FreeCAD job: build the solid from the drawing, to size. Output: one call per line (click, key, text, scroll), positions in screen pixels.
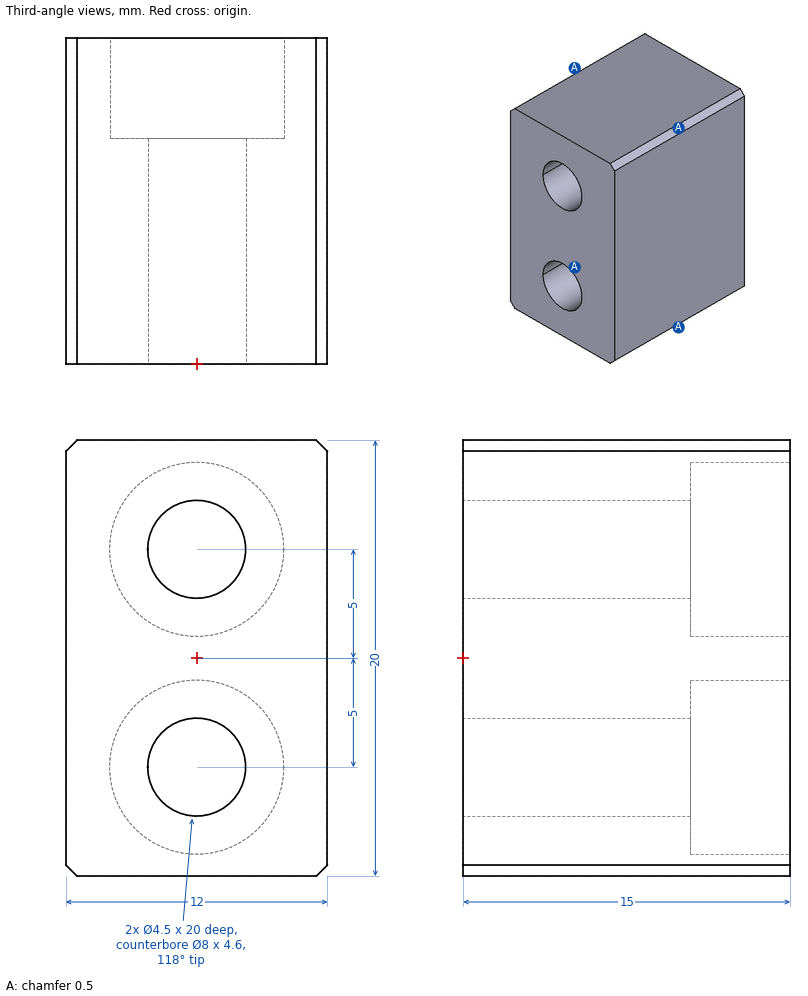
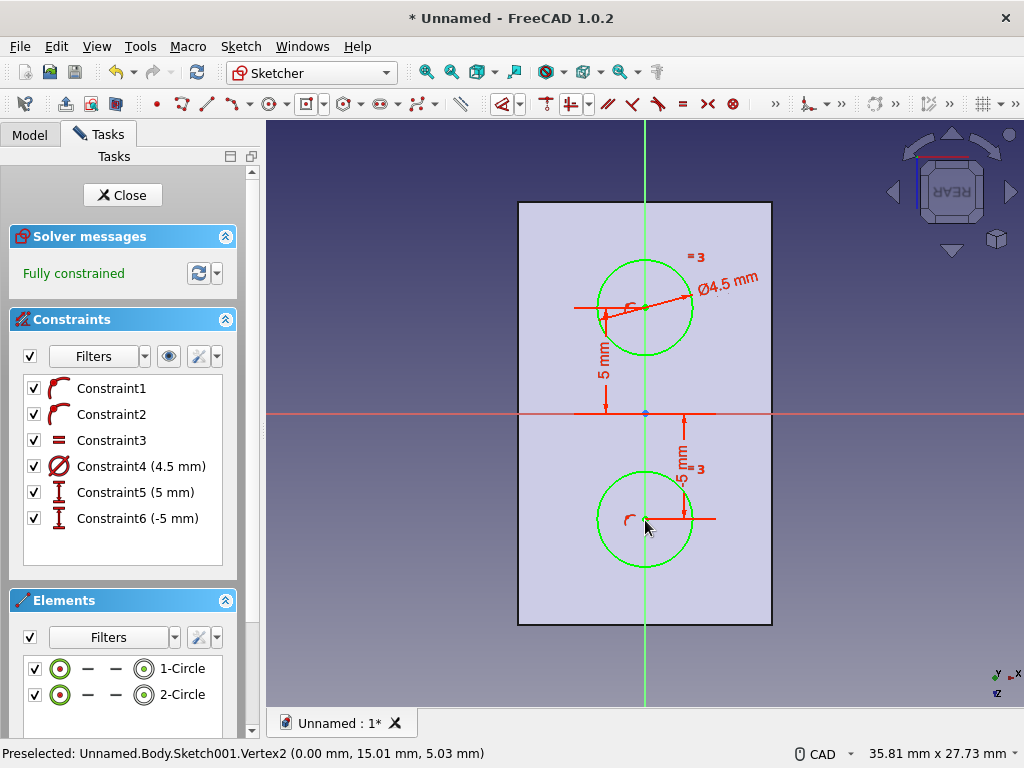
click(123, 195)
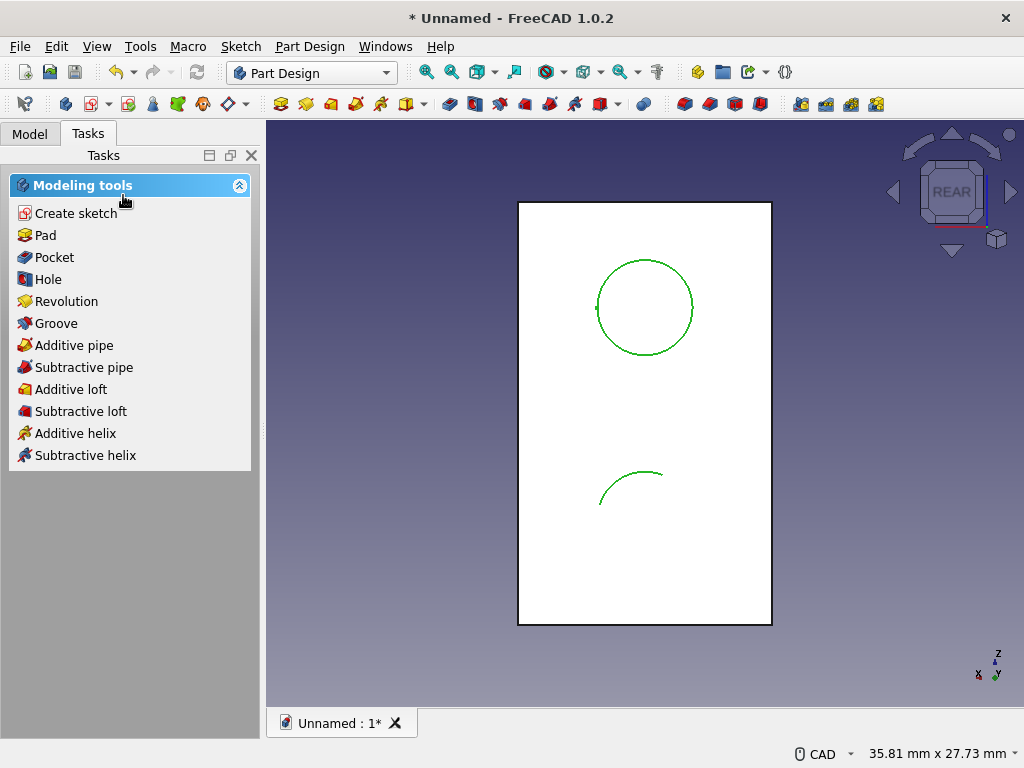
click(475, 104)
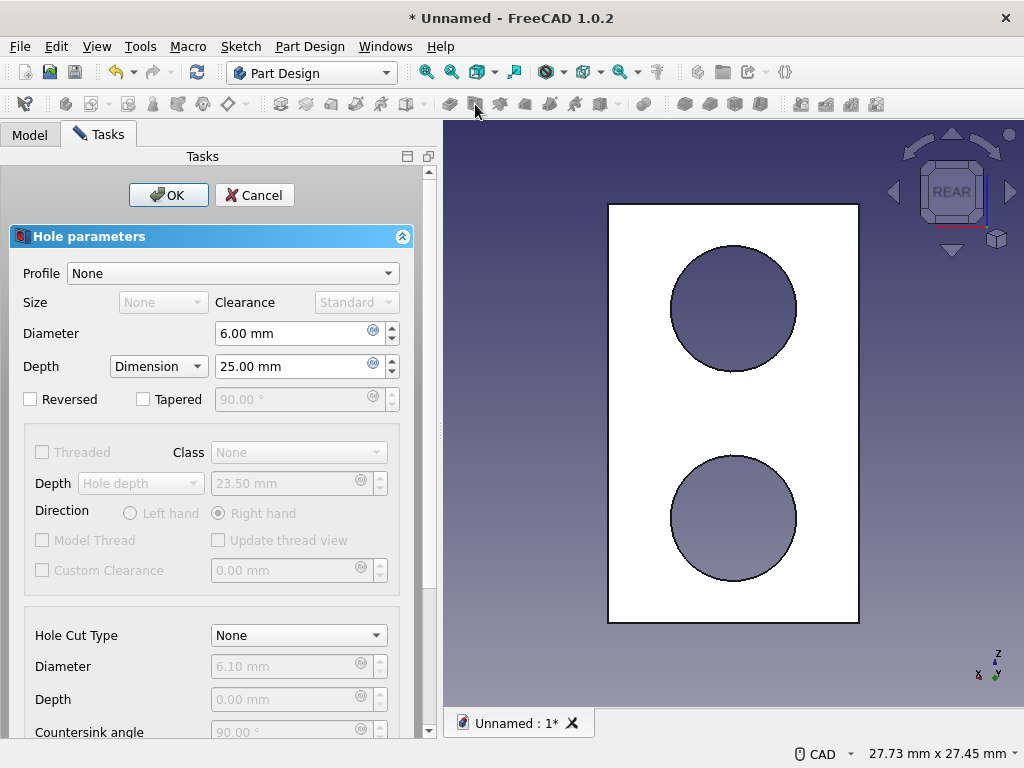
triple_click(300, 334)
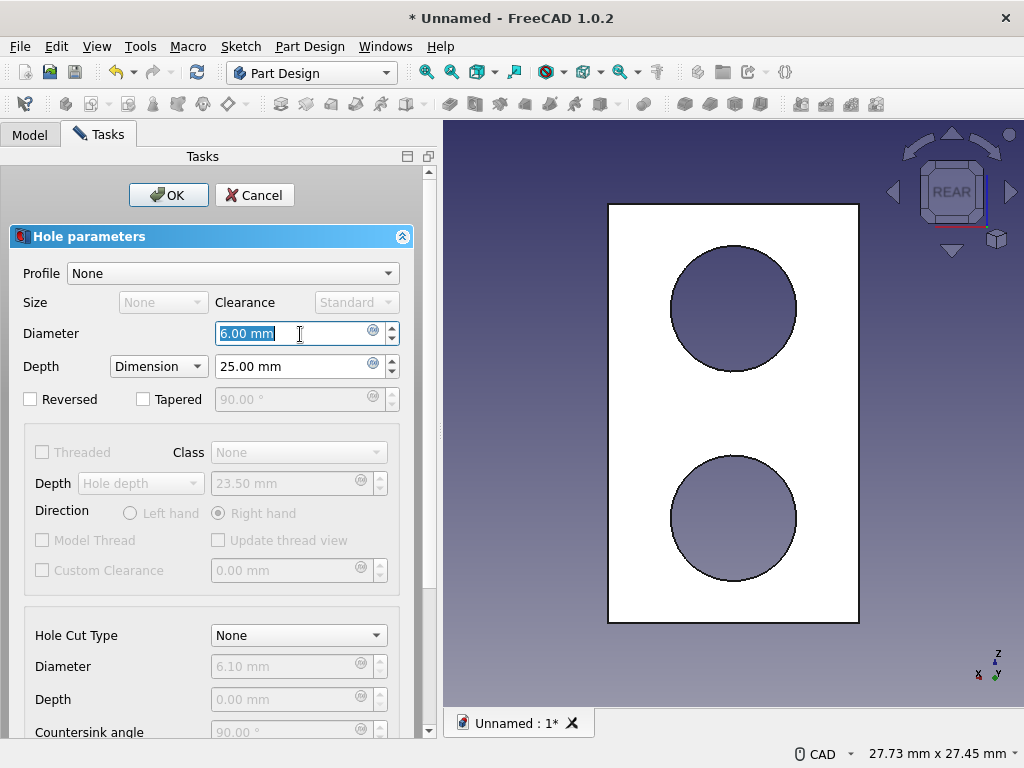
text(4.5)
key(Tab)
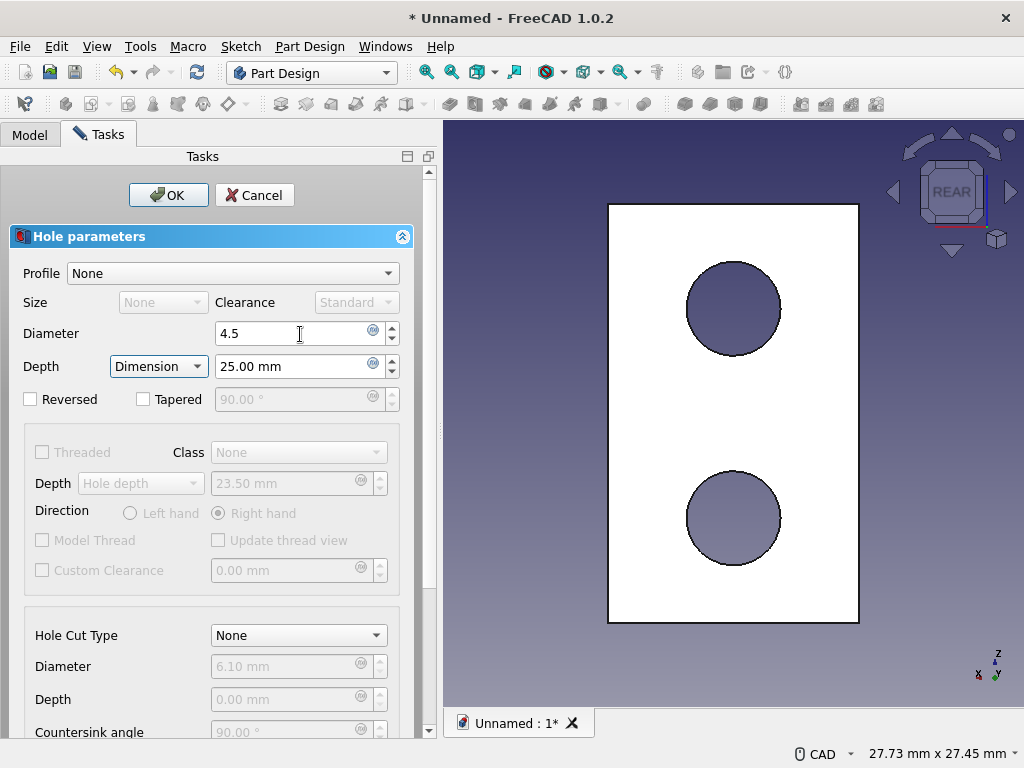
triple_click(300, 366)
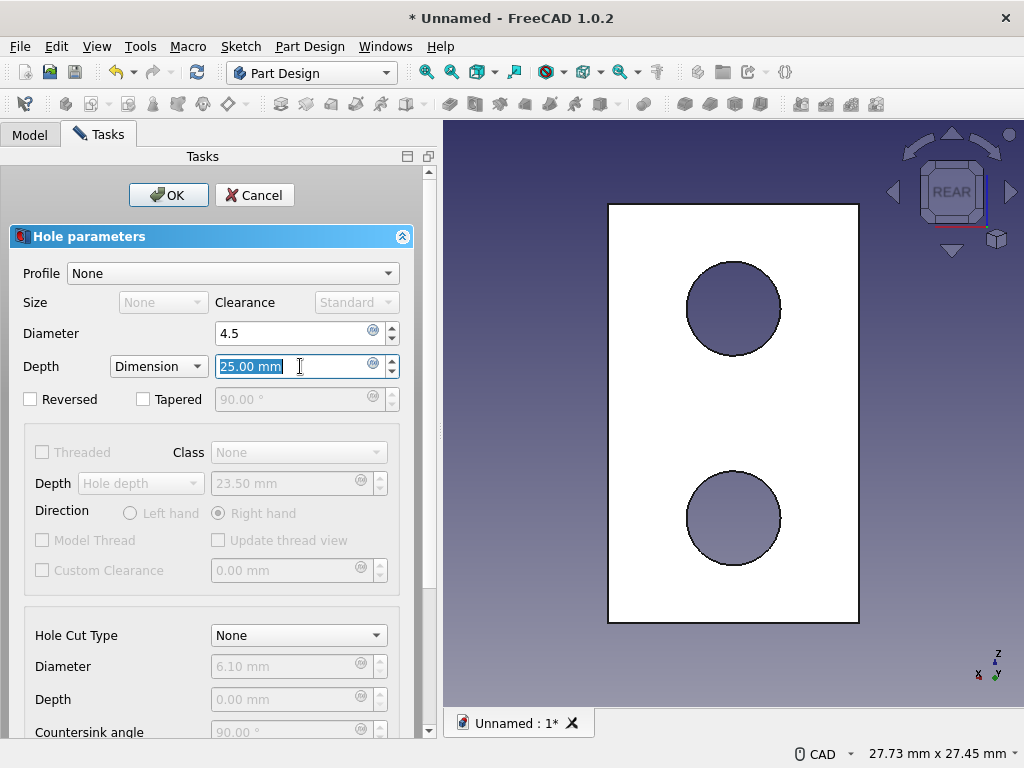
text(20)
key(Tab)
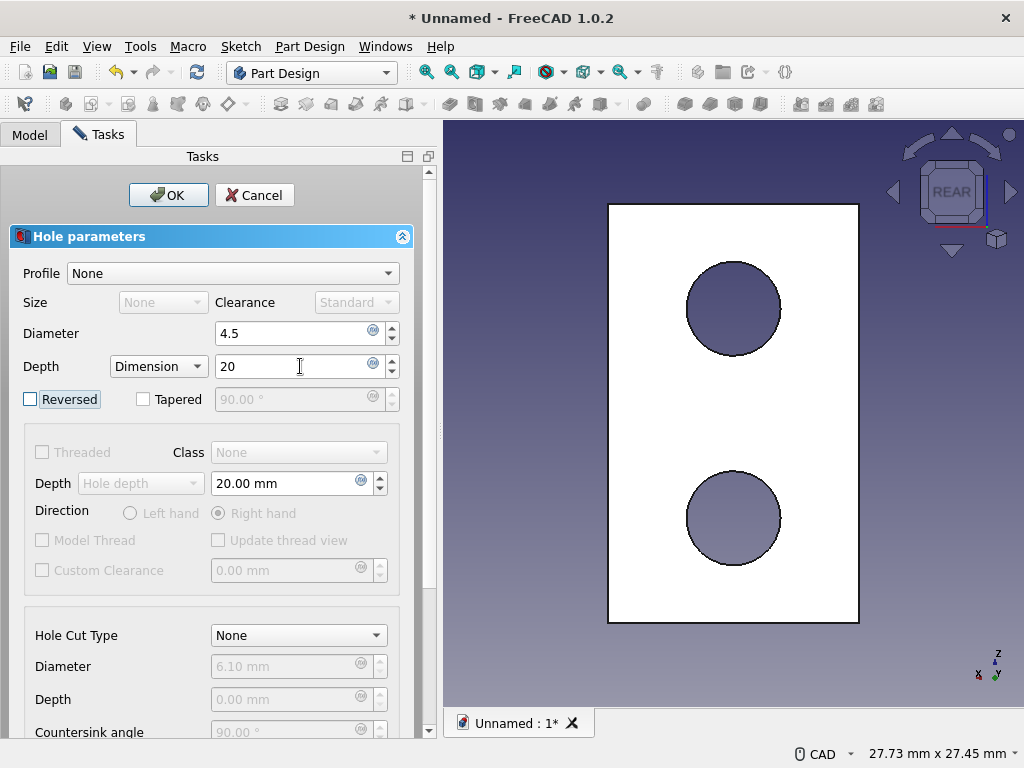
click(300, 636)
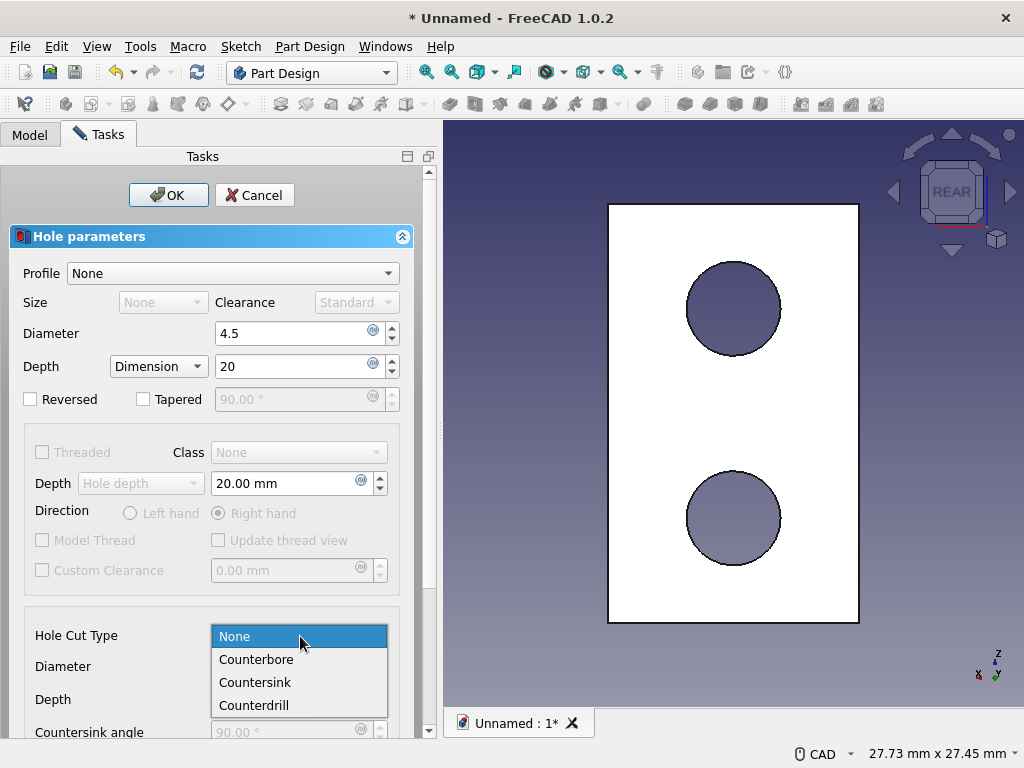
click(298, 660)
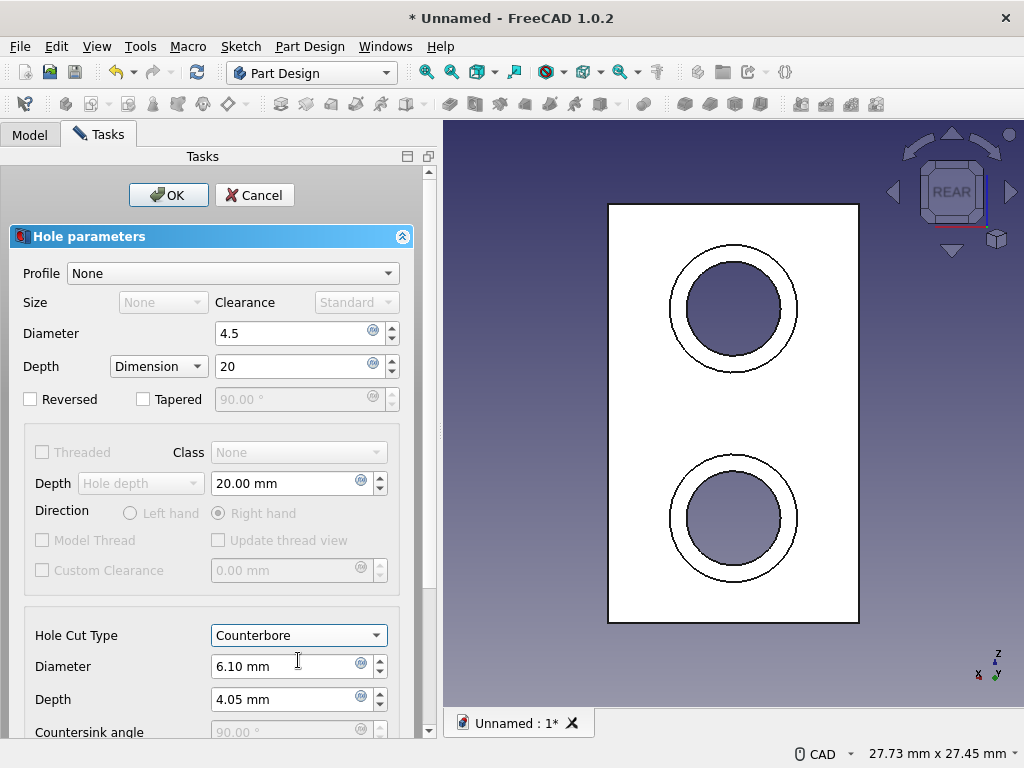
triple_click(292, 666)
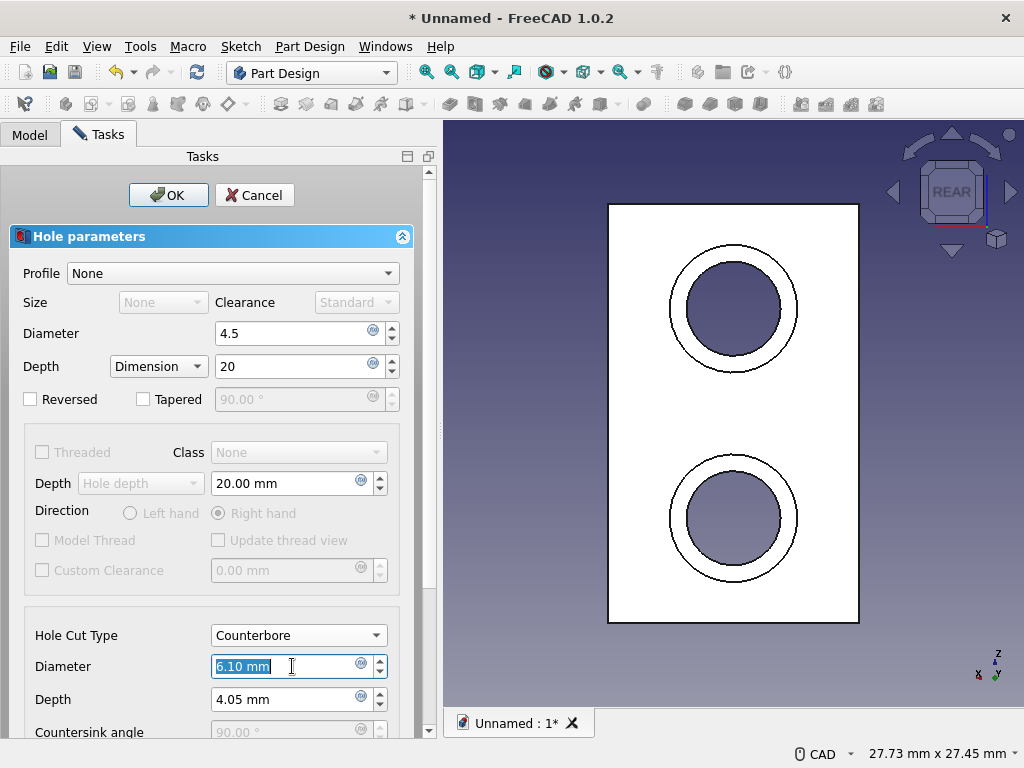
text(8)
key(Tab)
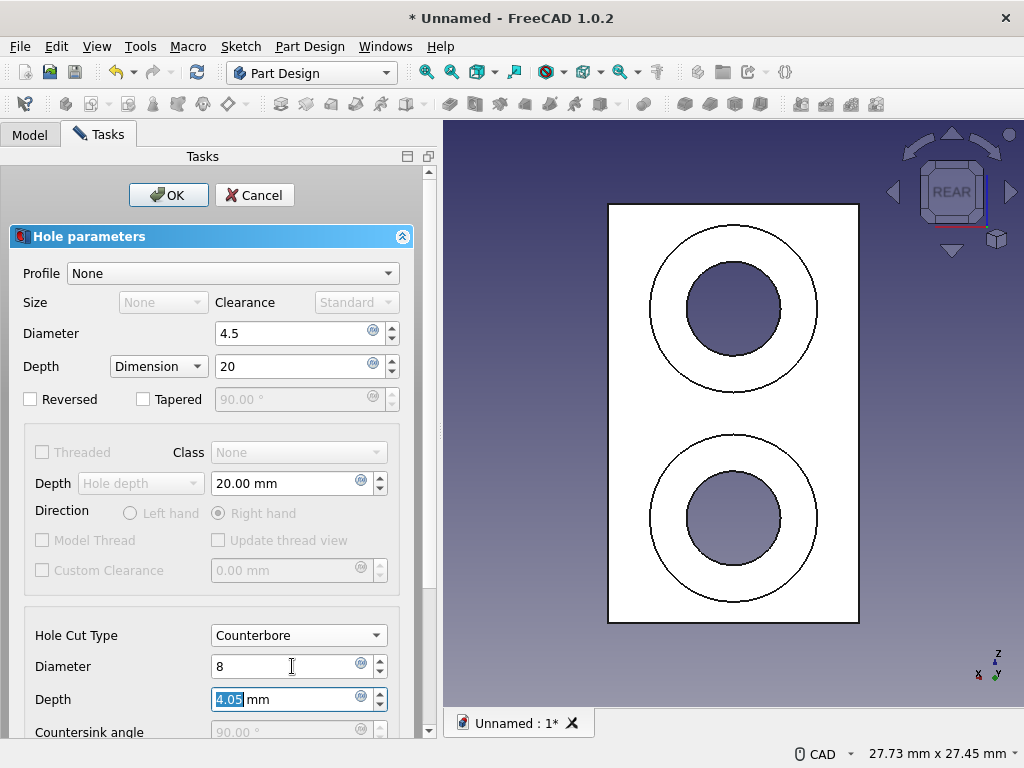
text(4.6)
key(Tab)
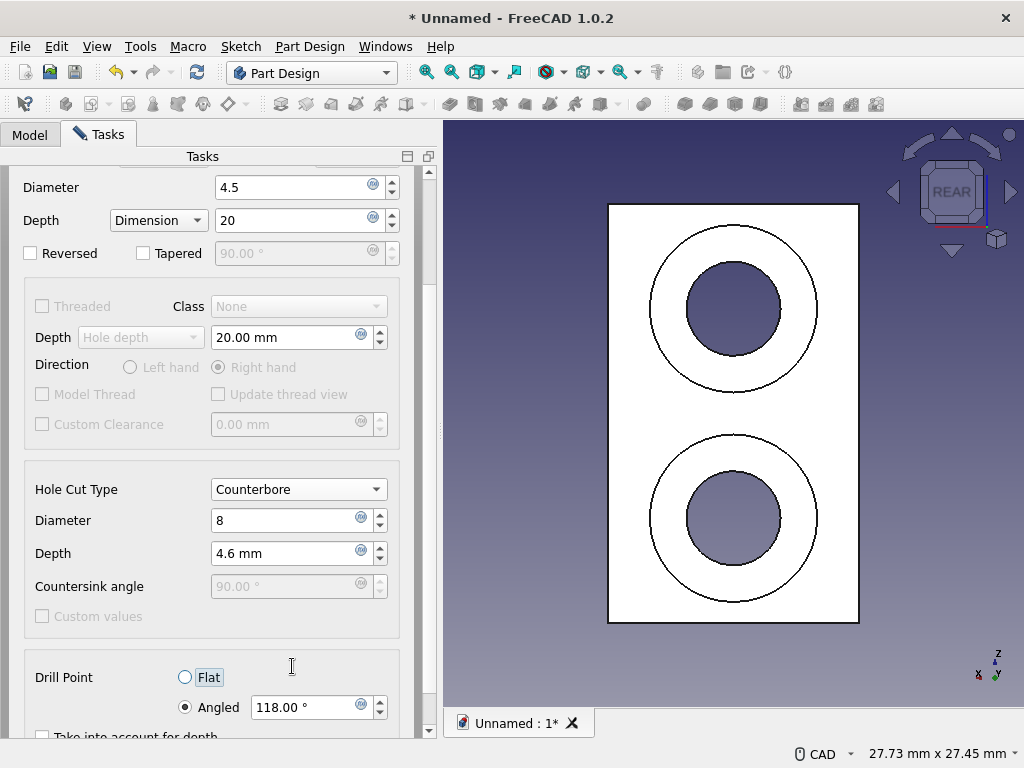
scroll(429, 452, up, 4)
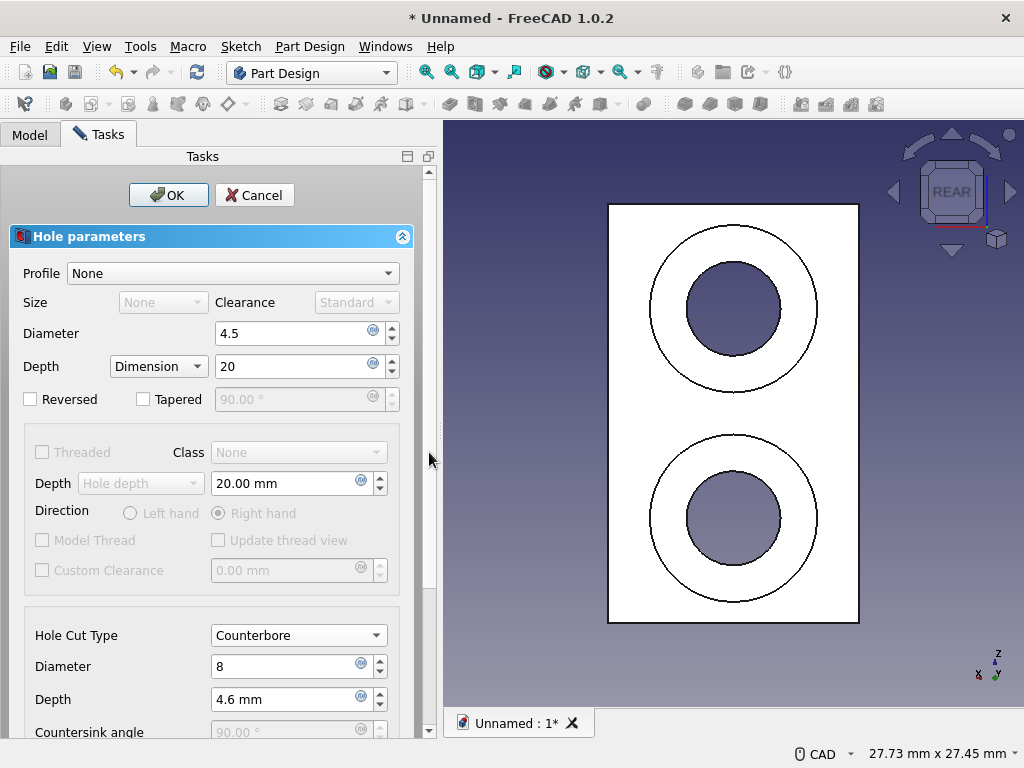
click(169, 195)